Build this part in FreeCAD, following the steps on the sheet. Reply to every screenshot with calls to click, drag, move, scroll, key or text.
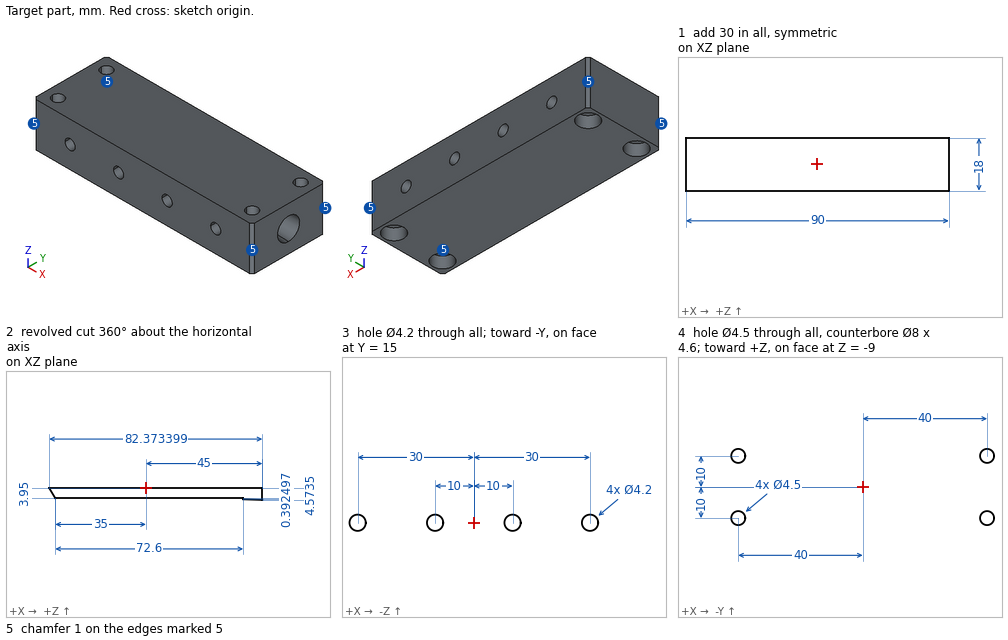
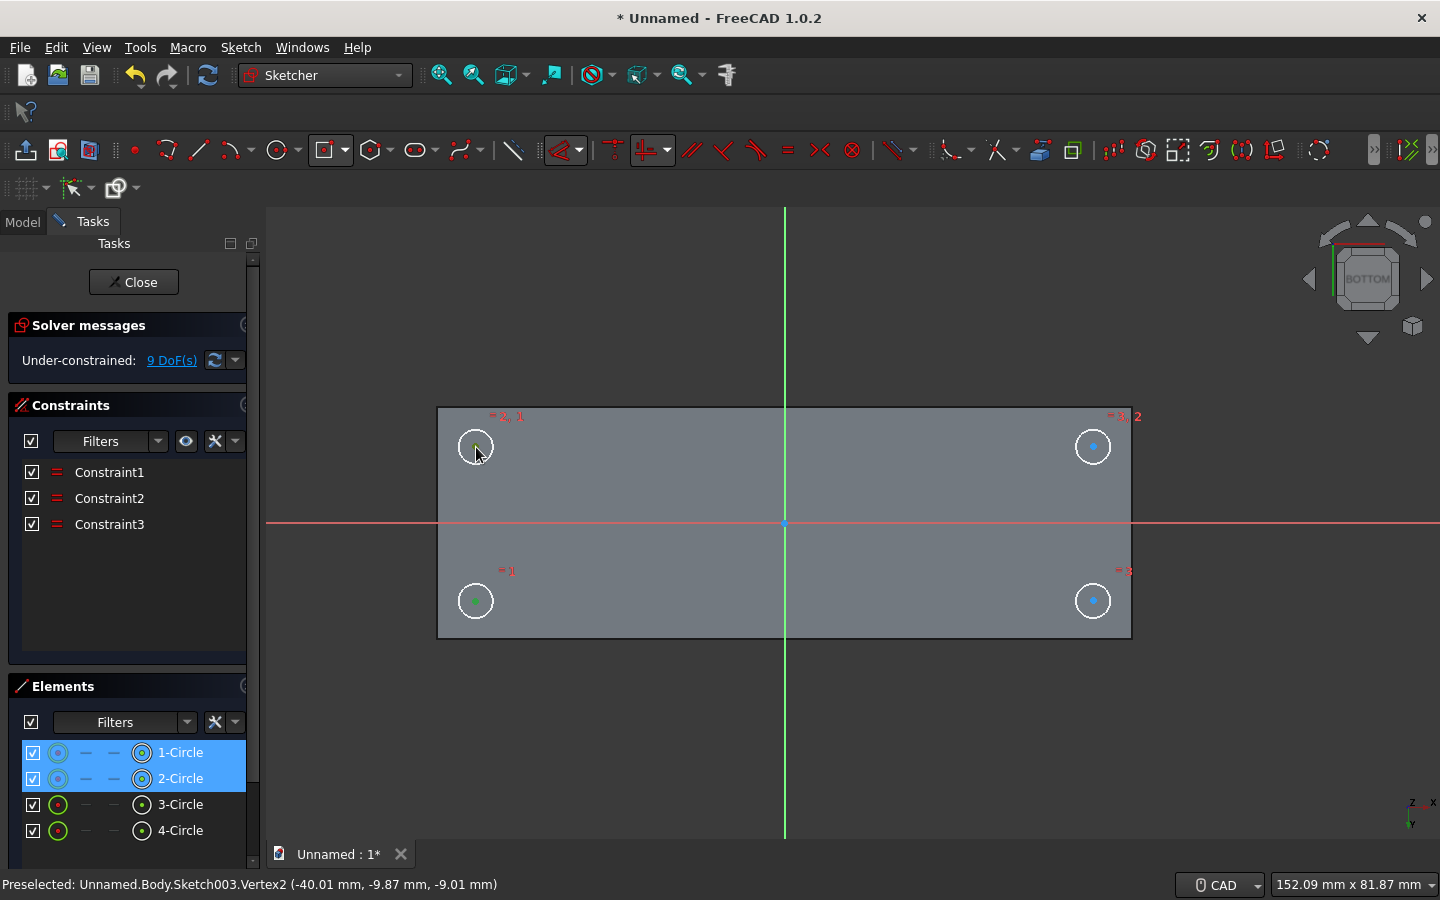
key(v)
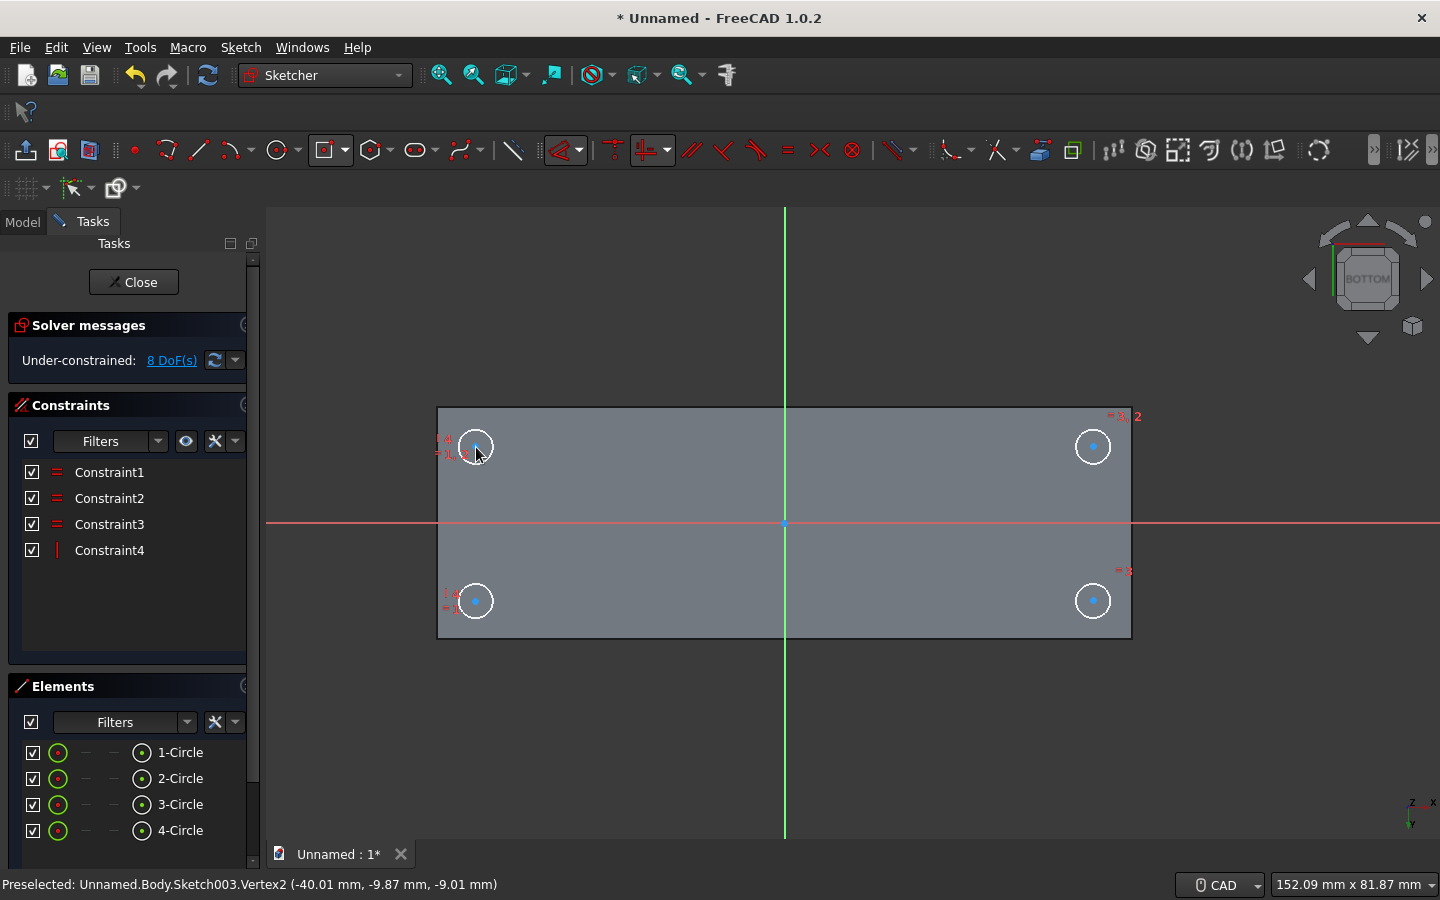
click(476, 447)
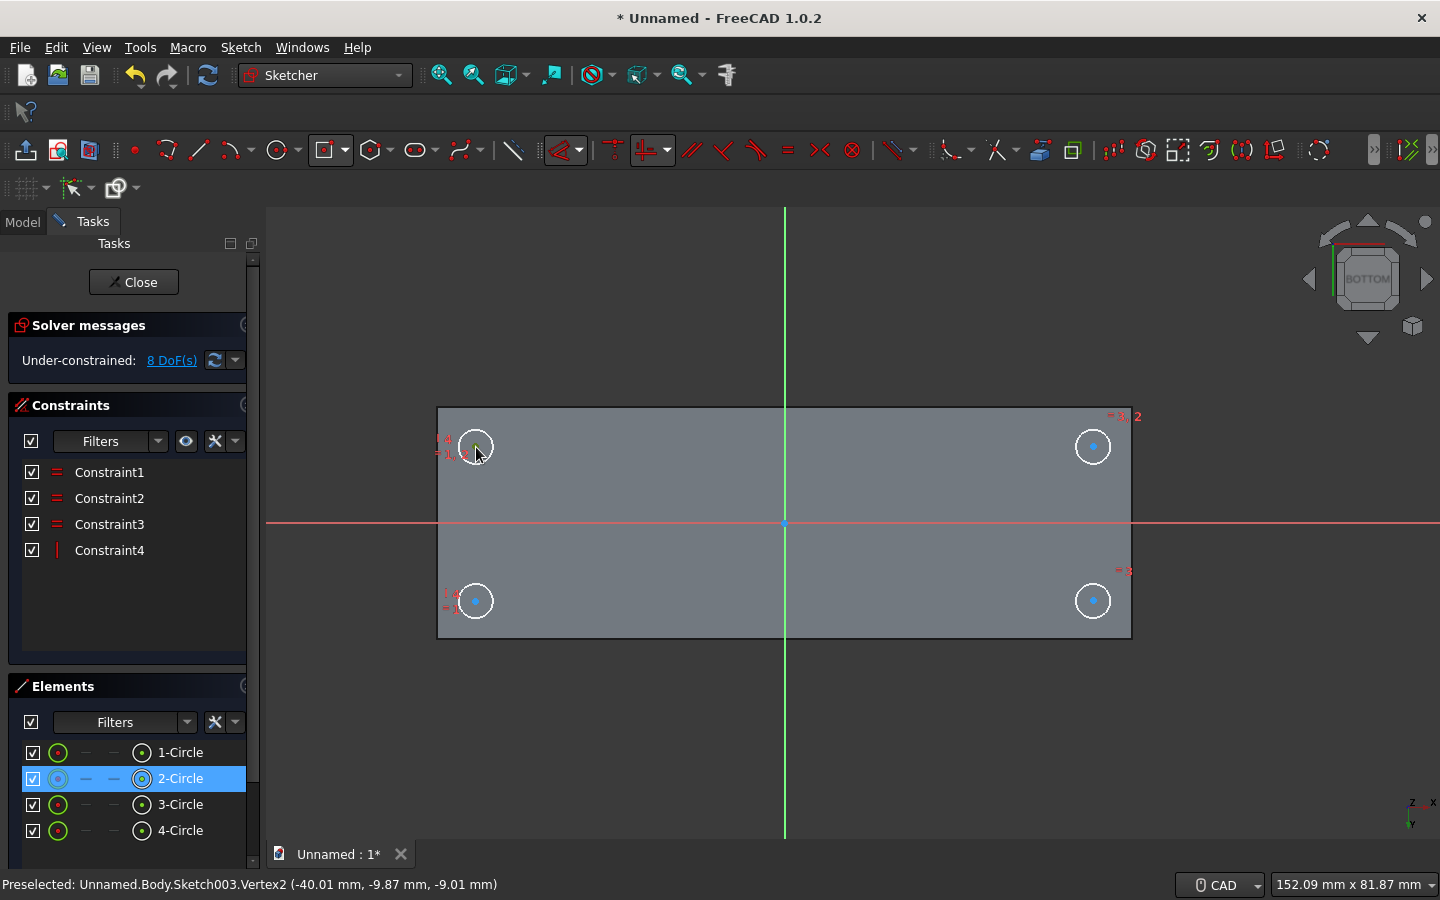
click(1093, 447)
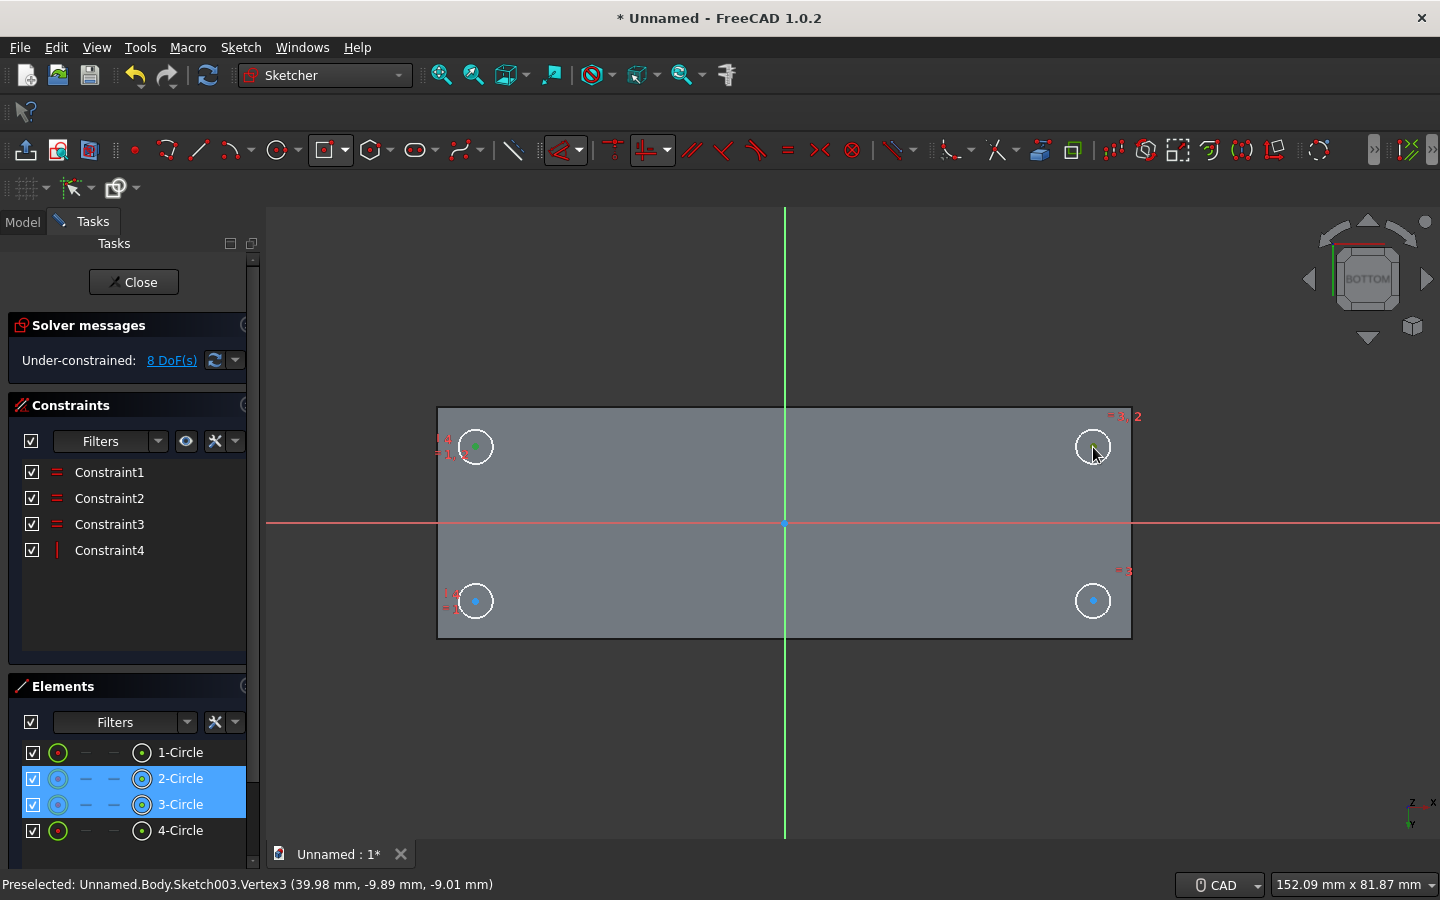
click(670, 150)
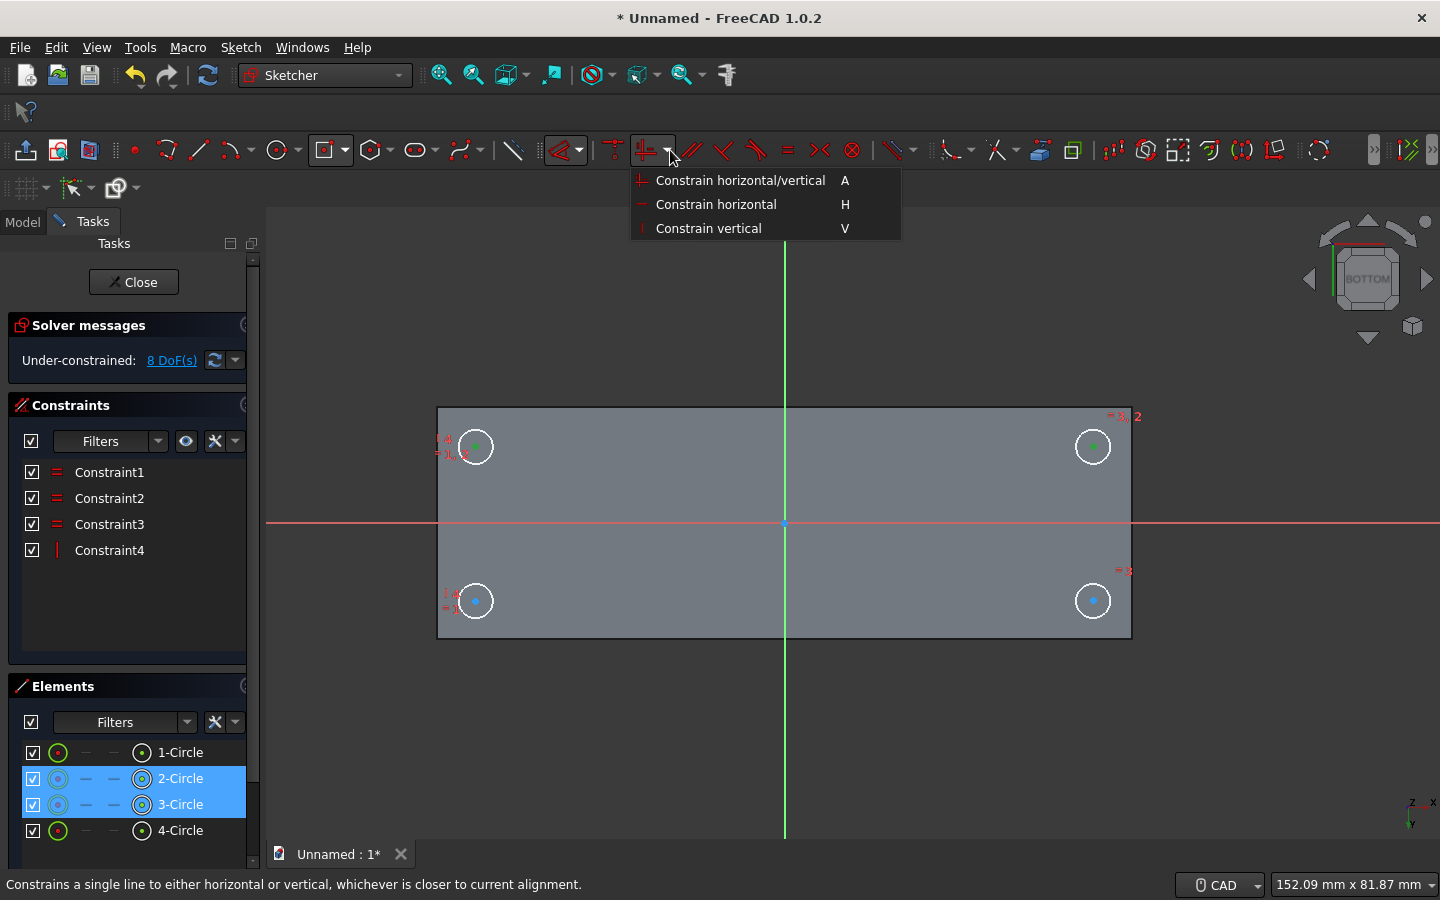
click(766, 204)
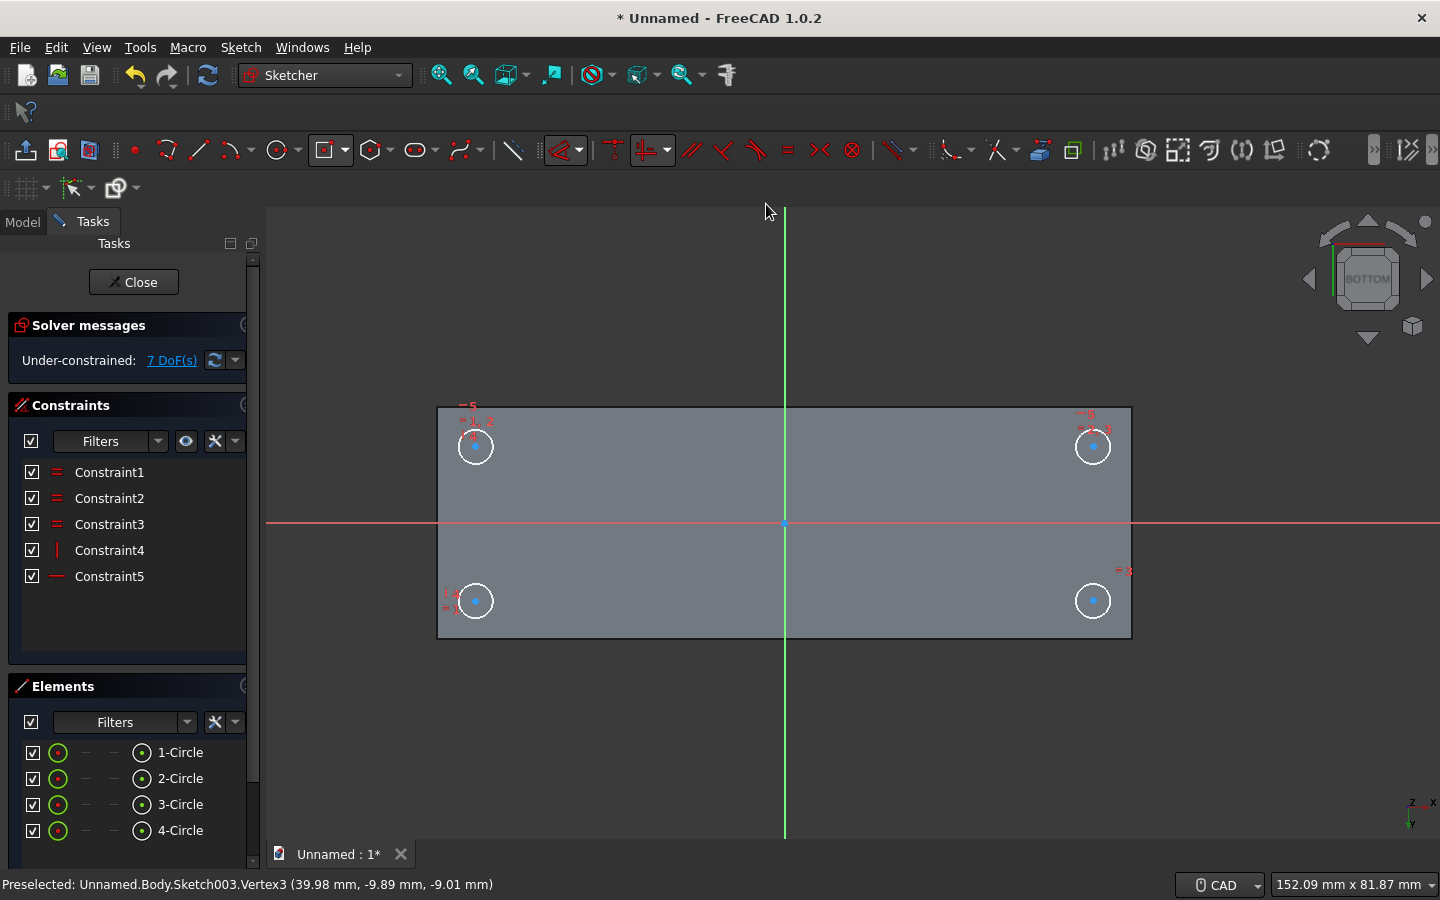
click(1093, 447)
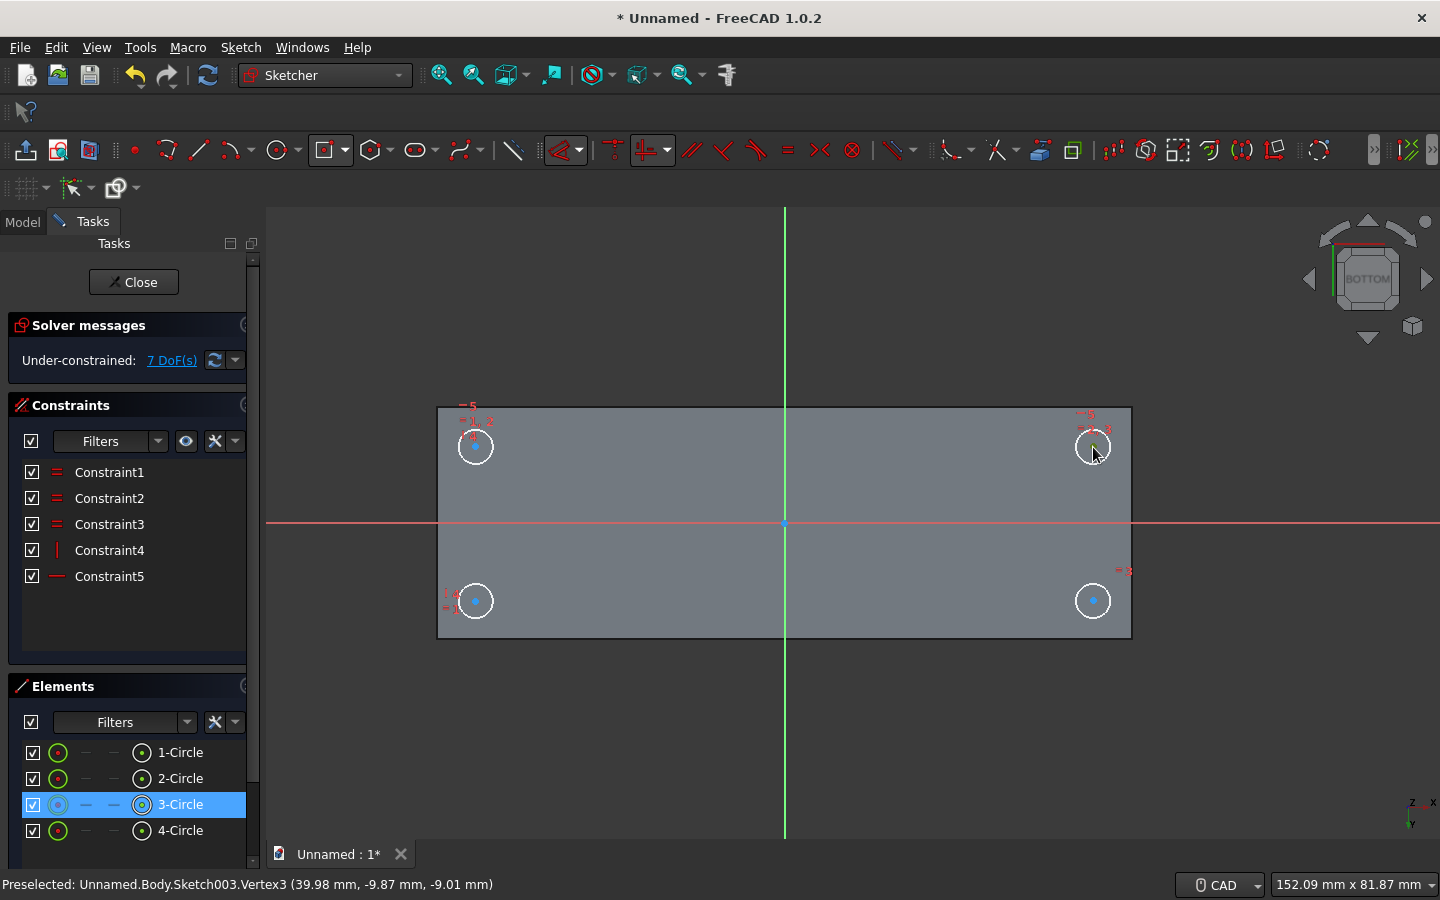
click(1093, 601)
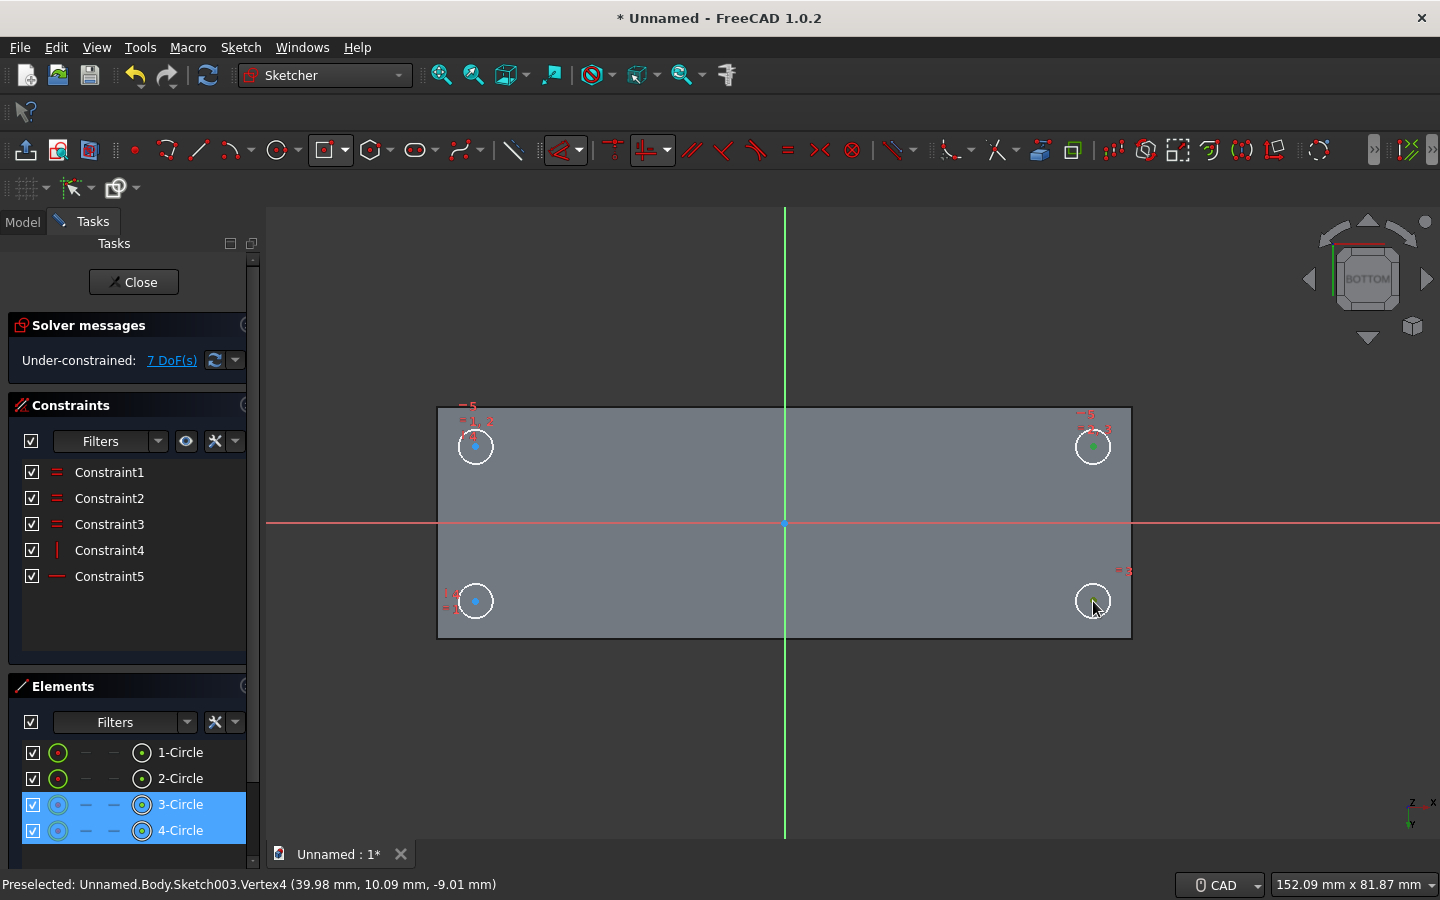
key(v)